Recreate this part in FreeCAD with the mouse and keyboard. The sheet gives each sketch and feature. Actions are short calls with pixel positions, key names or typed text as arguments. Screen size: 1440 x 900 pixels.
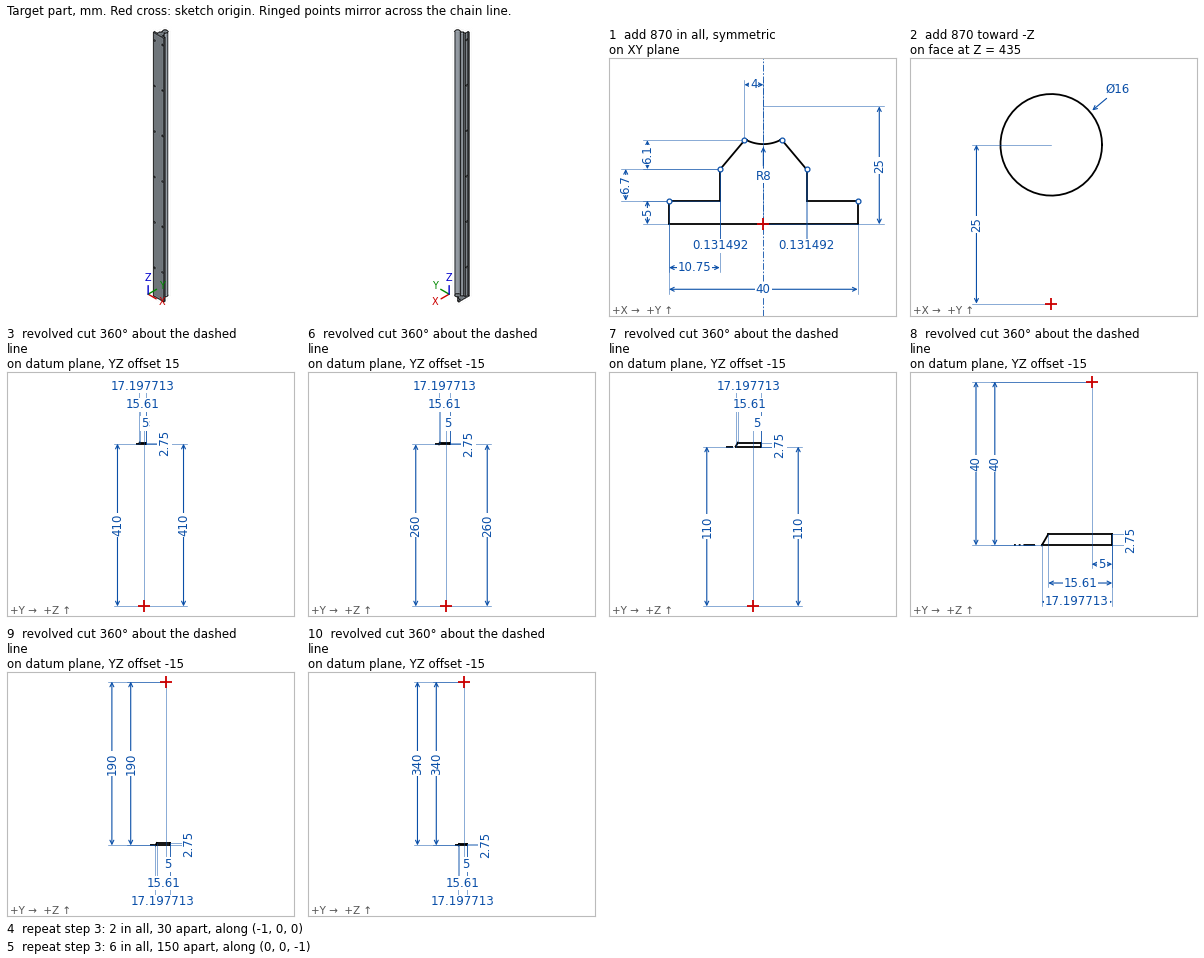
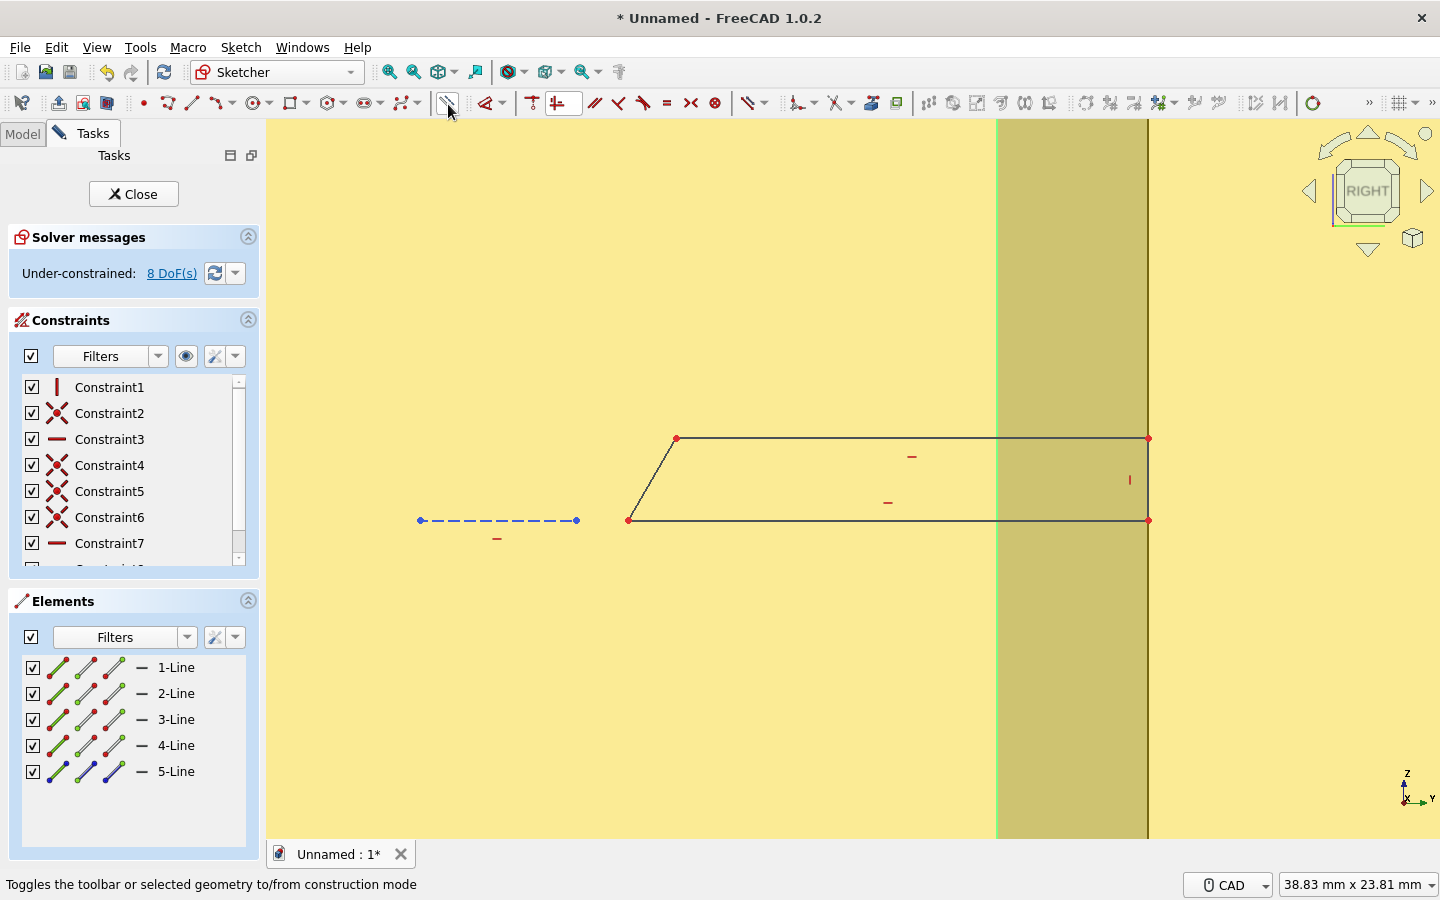
click(486, 104)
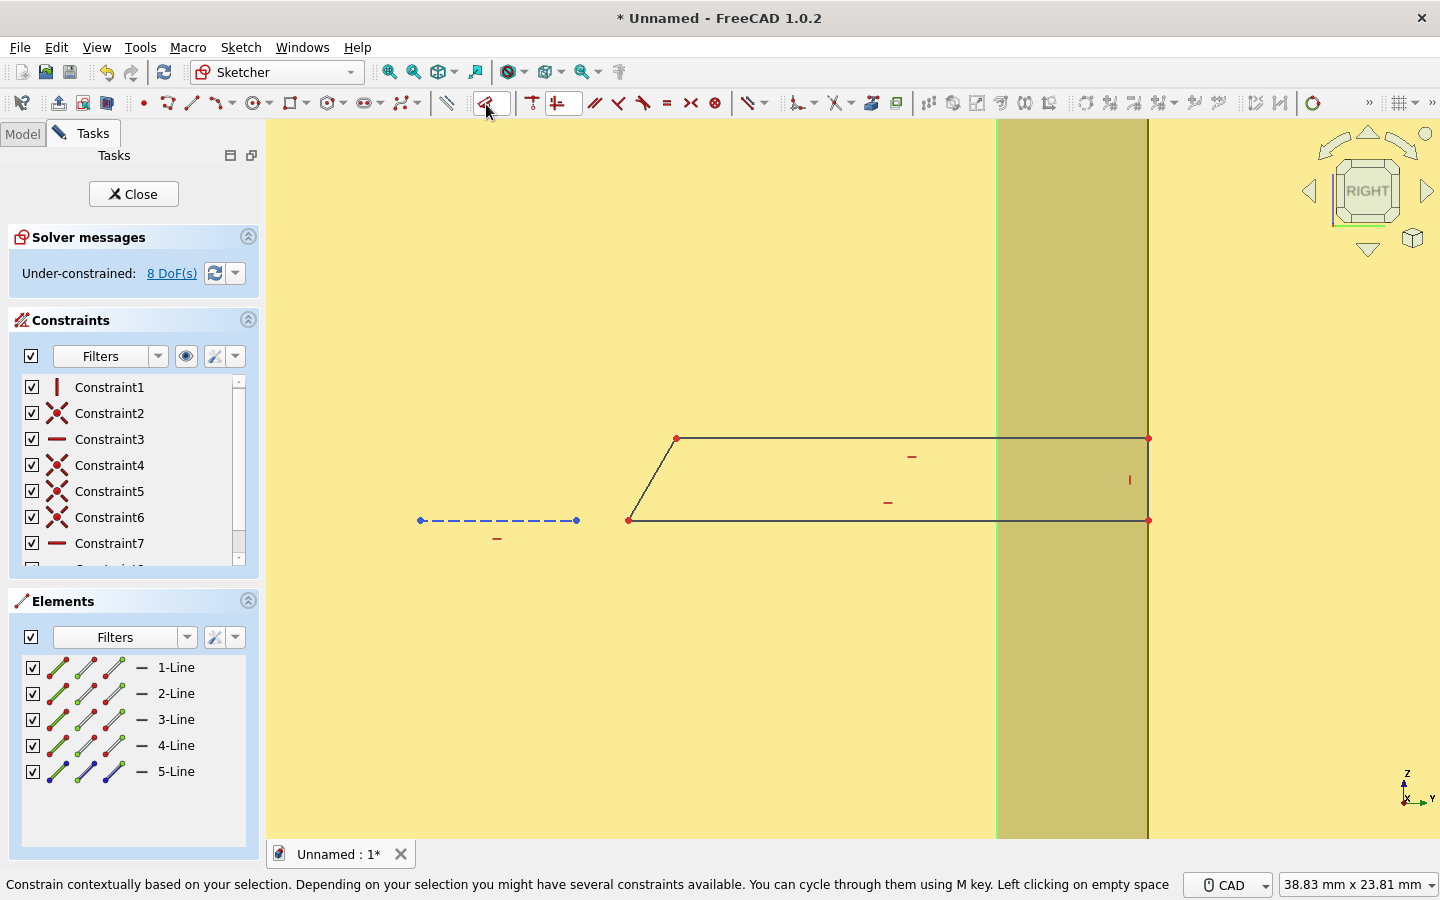
click(1148, 521)
click(1072, 487)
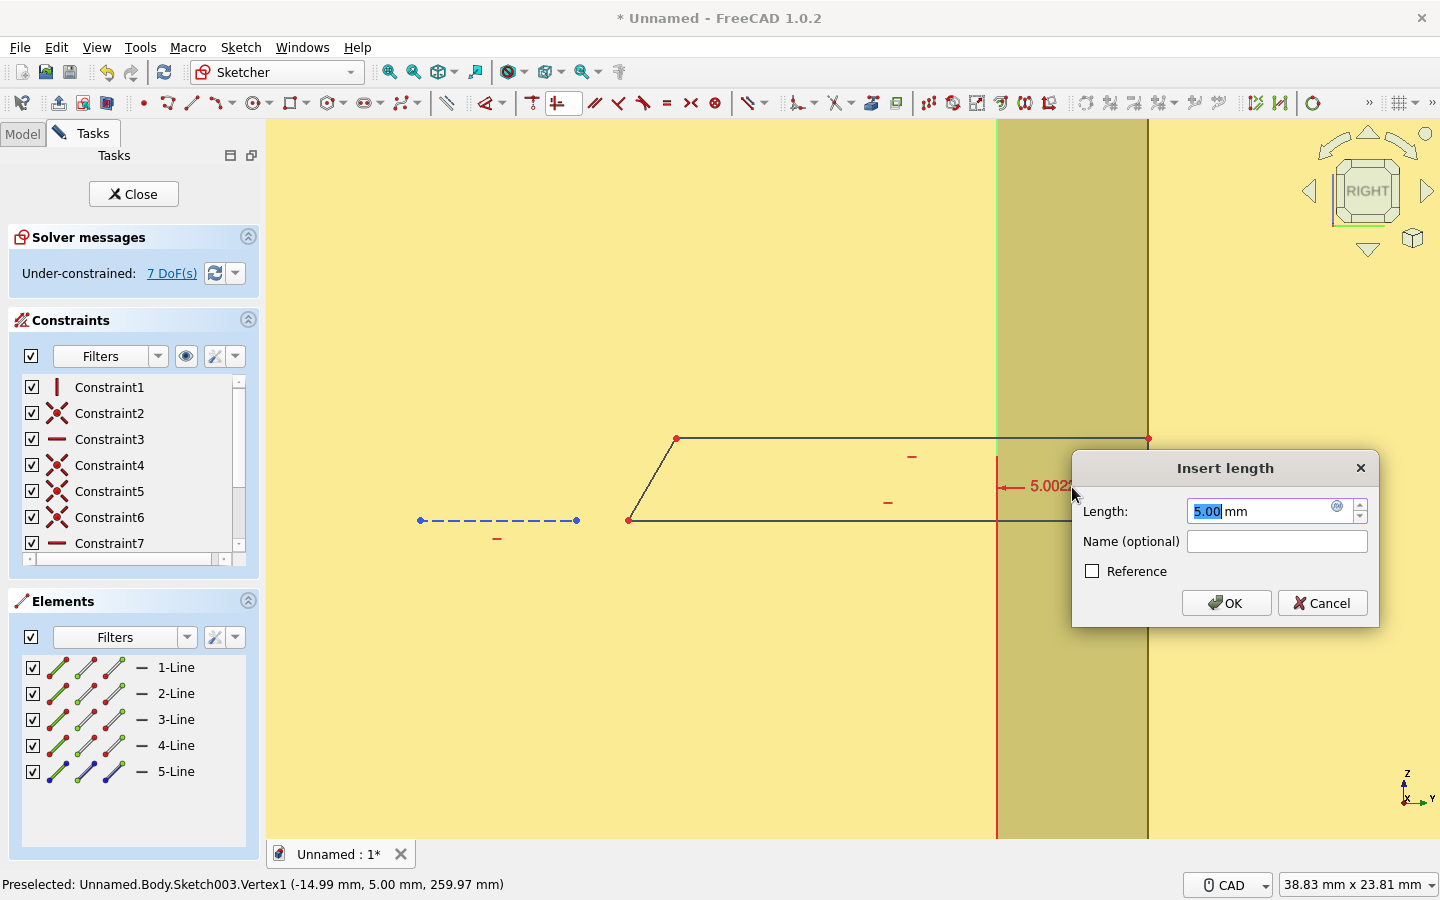
text(5)
key(Return)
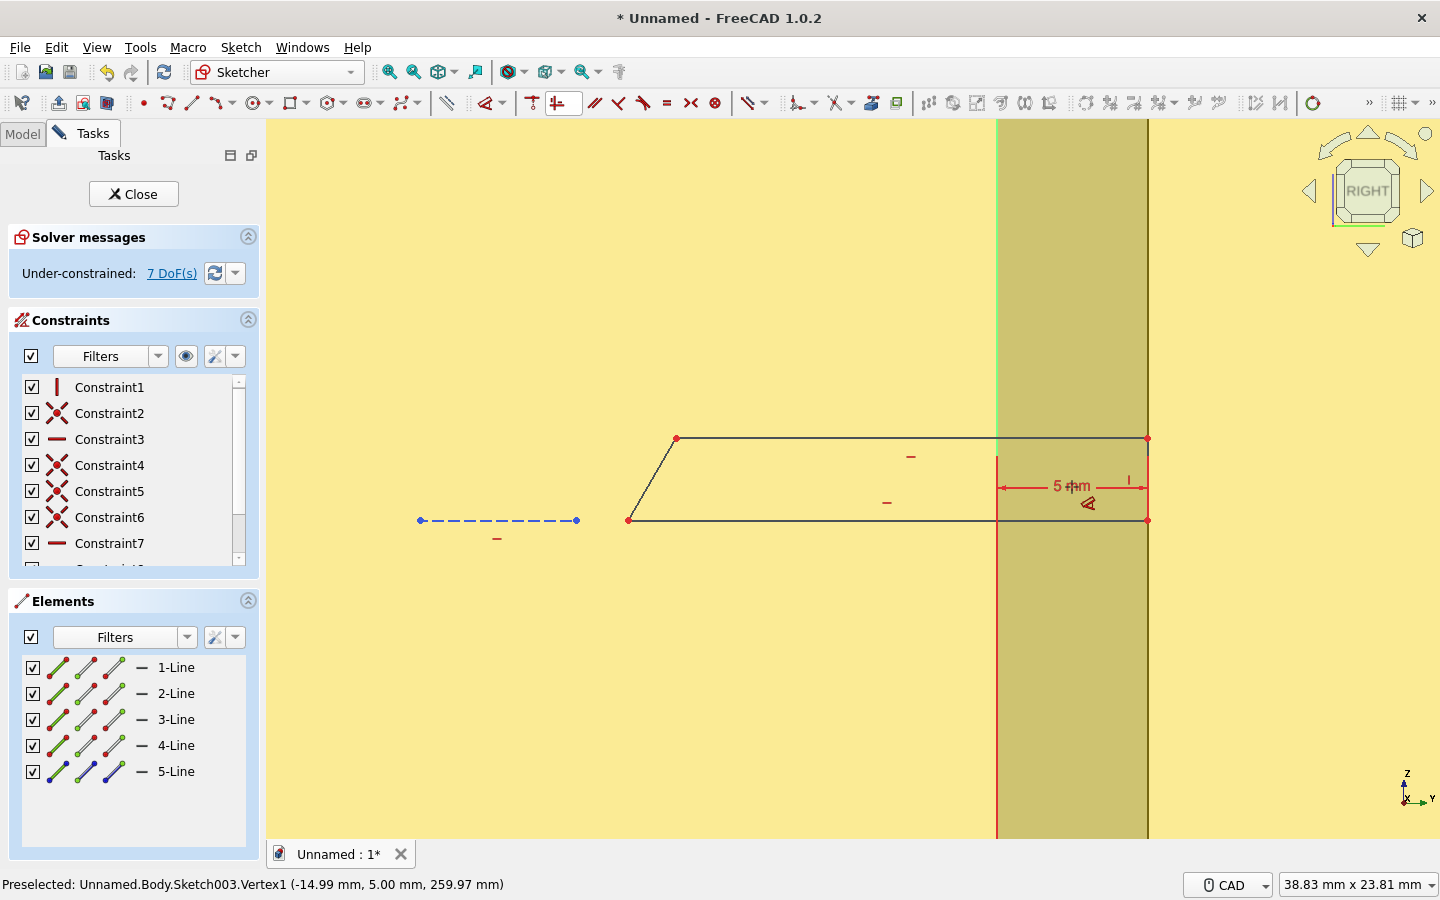
click(1148, 496)
click(1182, 480)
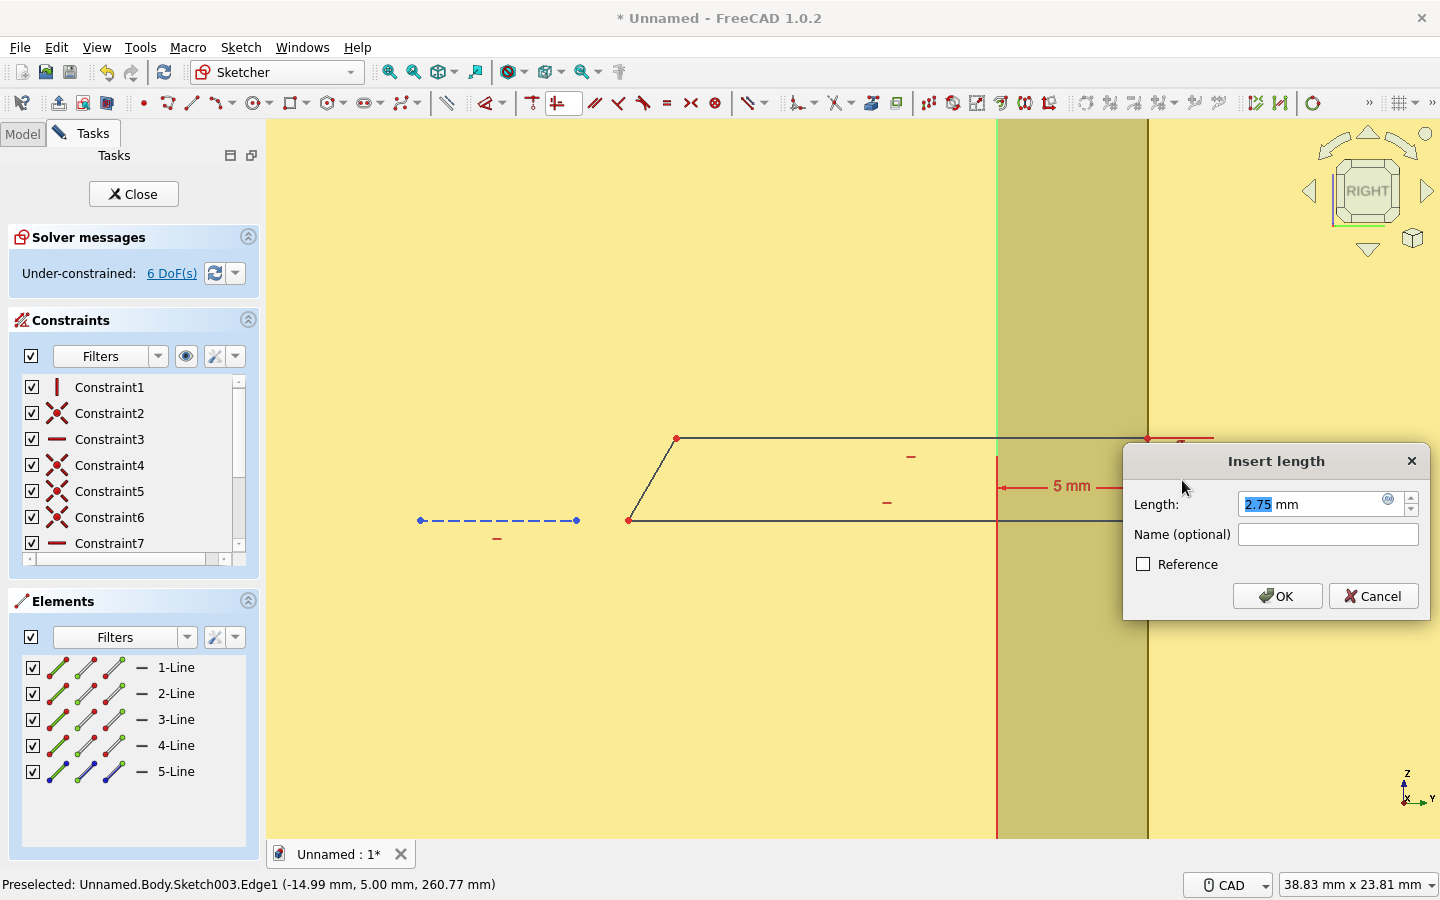
text(2.75)
key(Return)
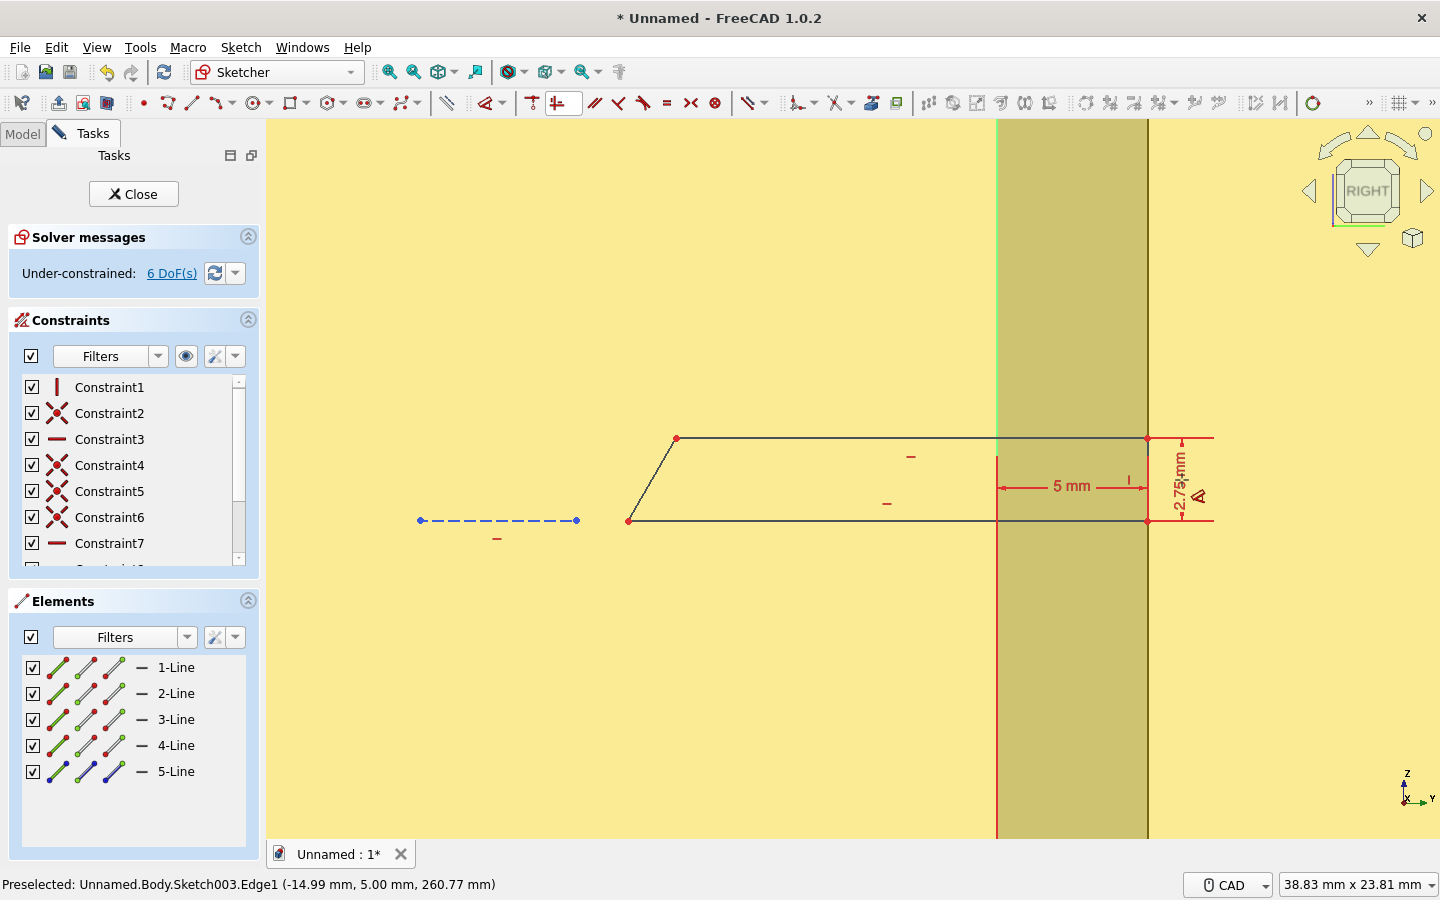
click(1148, 521)
click(1182, 666)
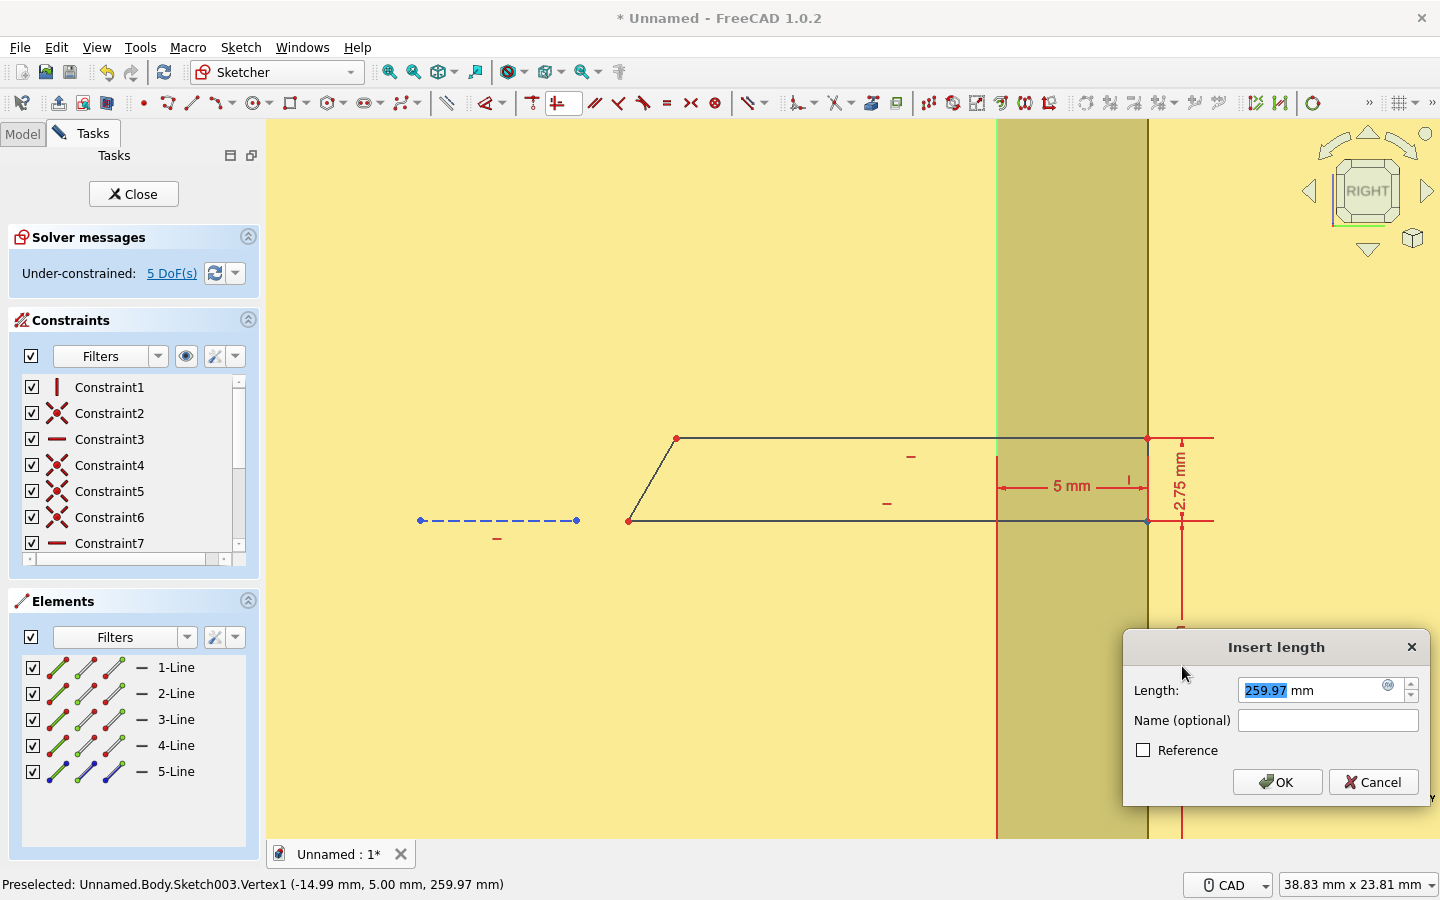
text(260)
key(Return)